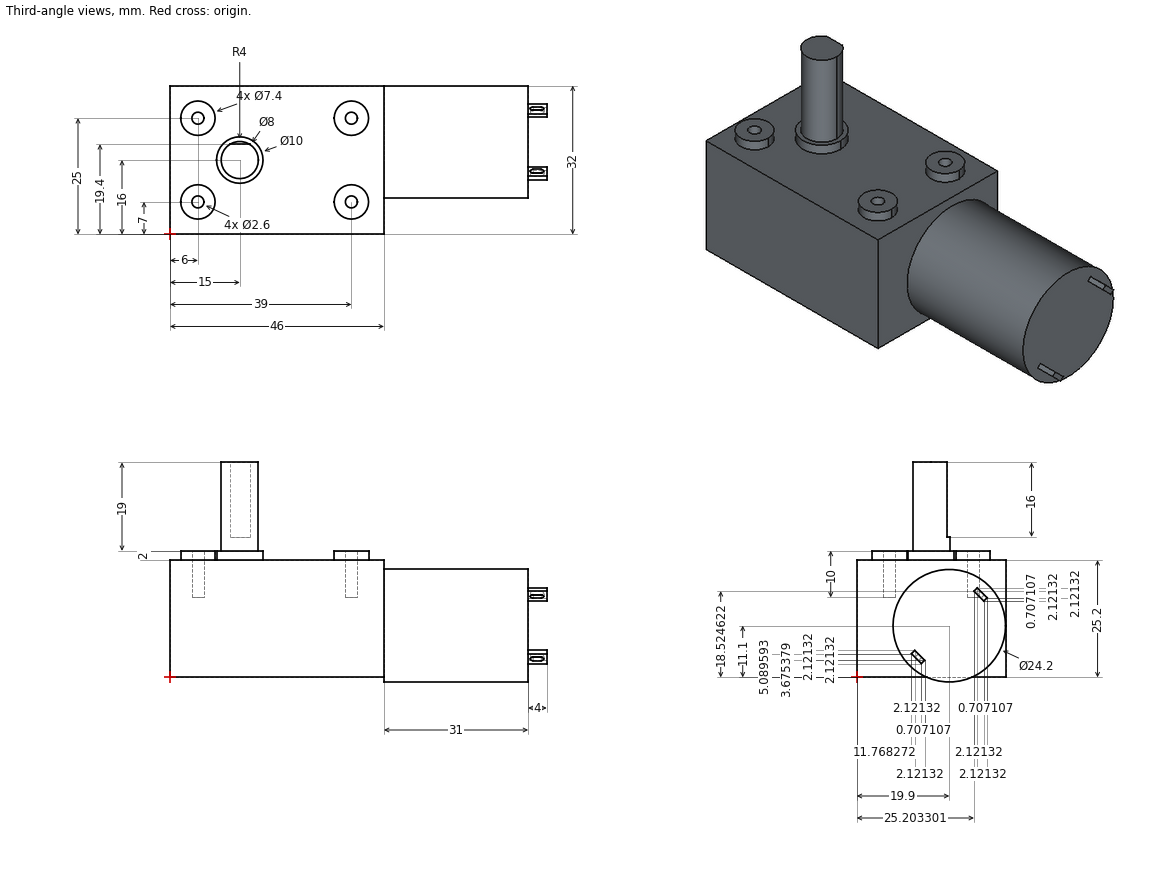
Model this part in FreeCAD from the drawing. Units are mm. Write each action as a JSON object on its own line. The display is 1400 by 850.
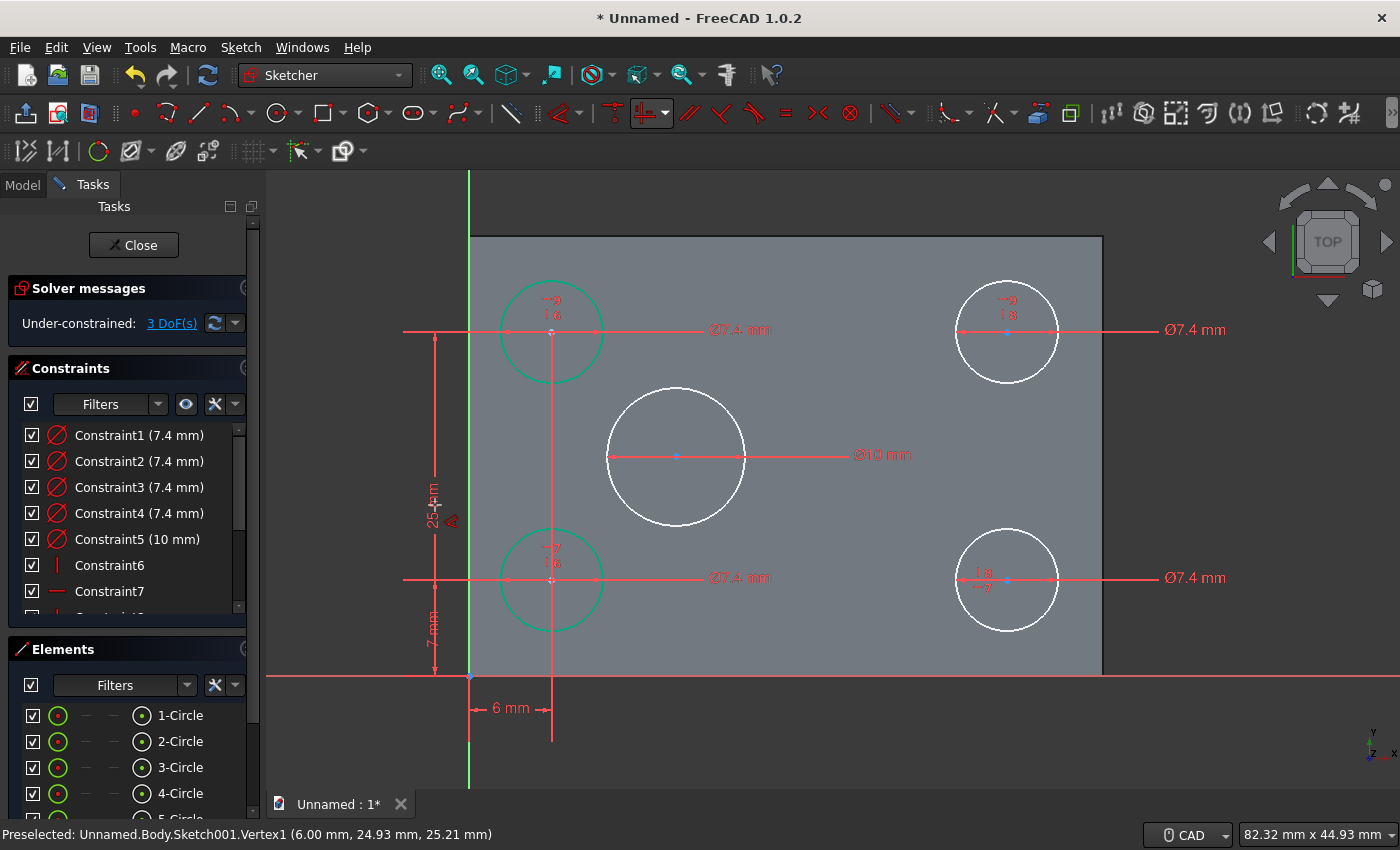
{"action": "left_click", "coordinate": [1007, 580]}
{"action": "left_click", "coordinate": [738, 710]}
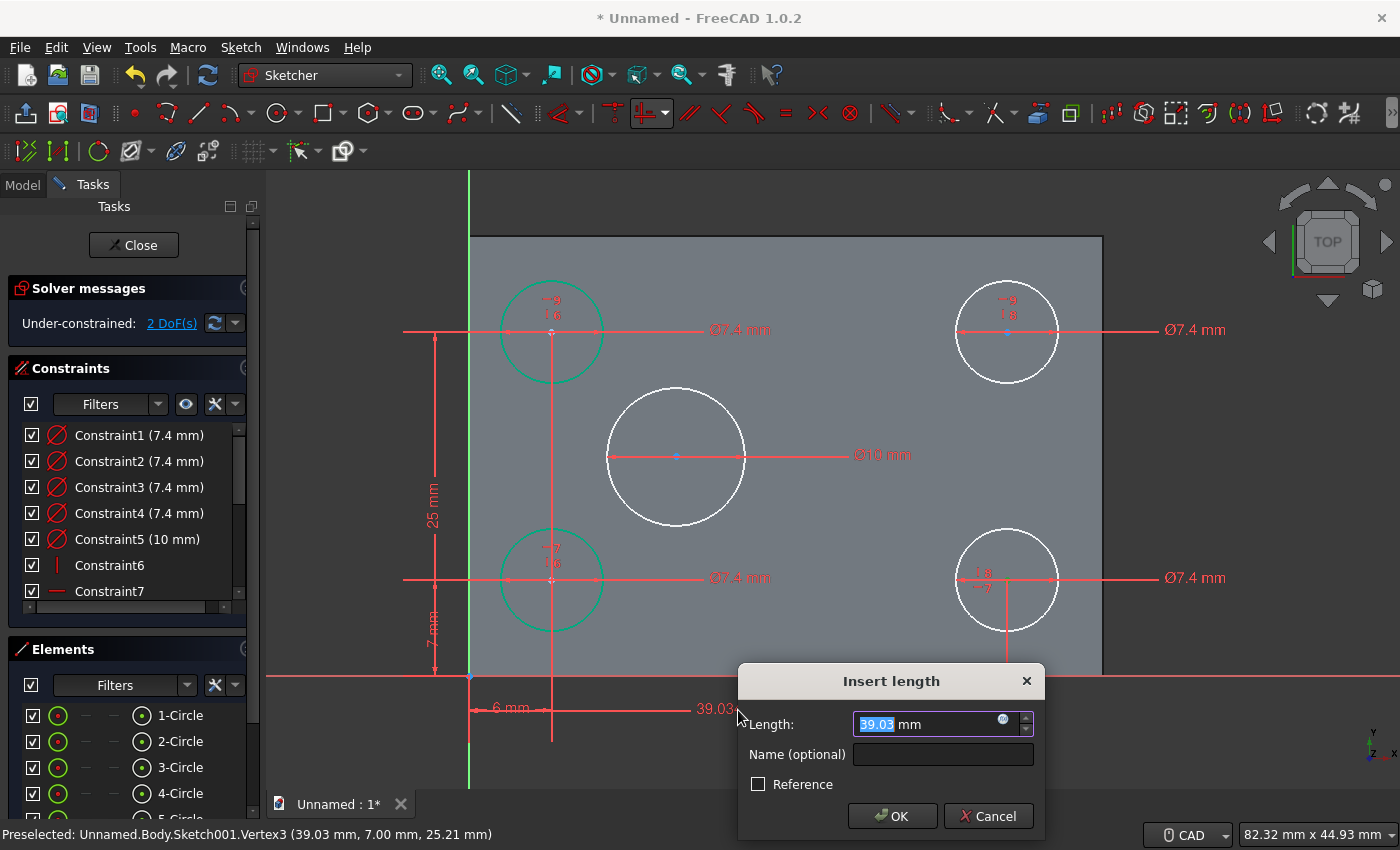
{"action": "type", "text": "39"}
{"action": "key", "text": "Return"}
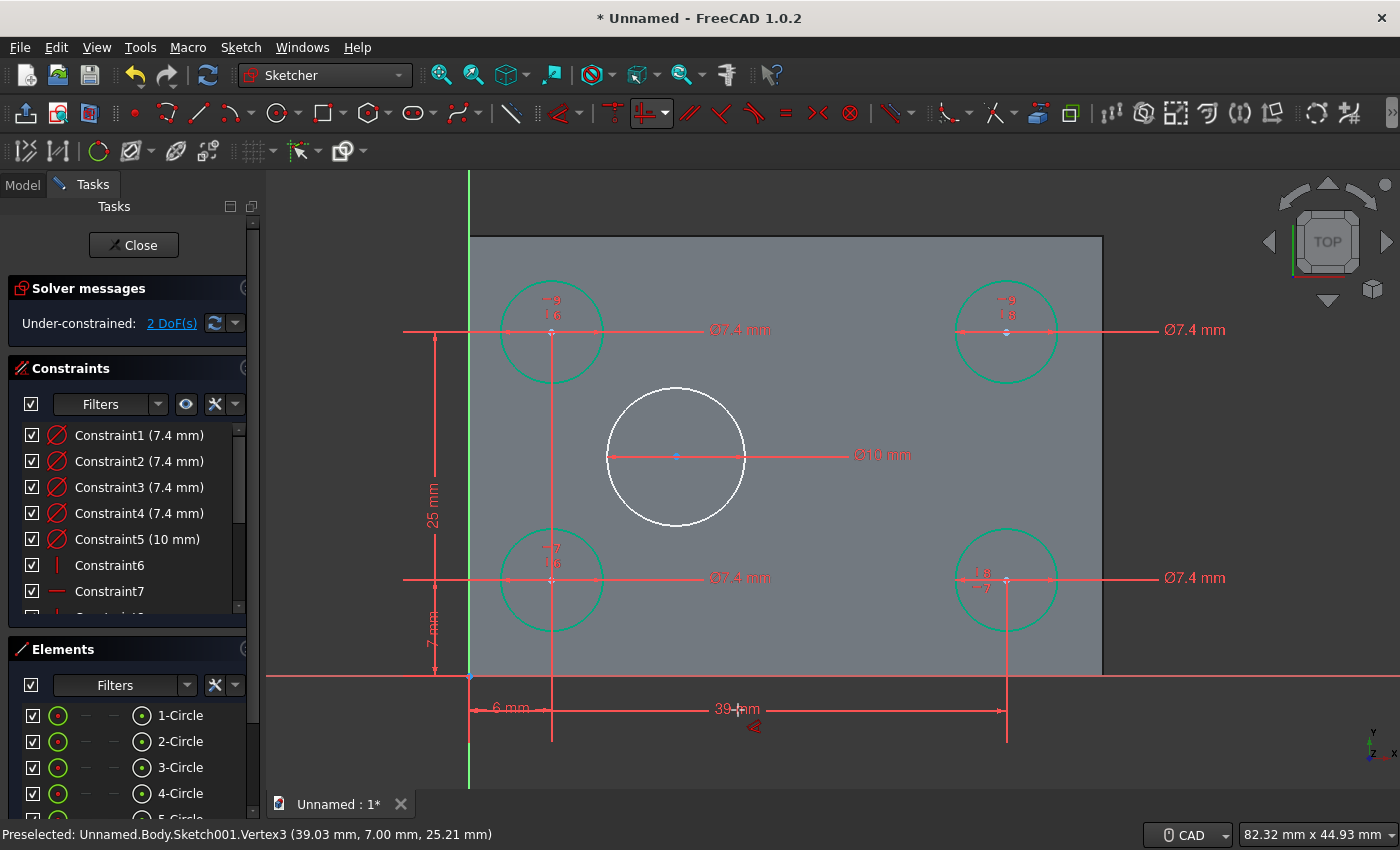
{"action": "left_click", "coordinate": [676, 457]}
{"action": "left_click", "coordinate": [620, 710]}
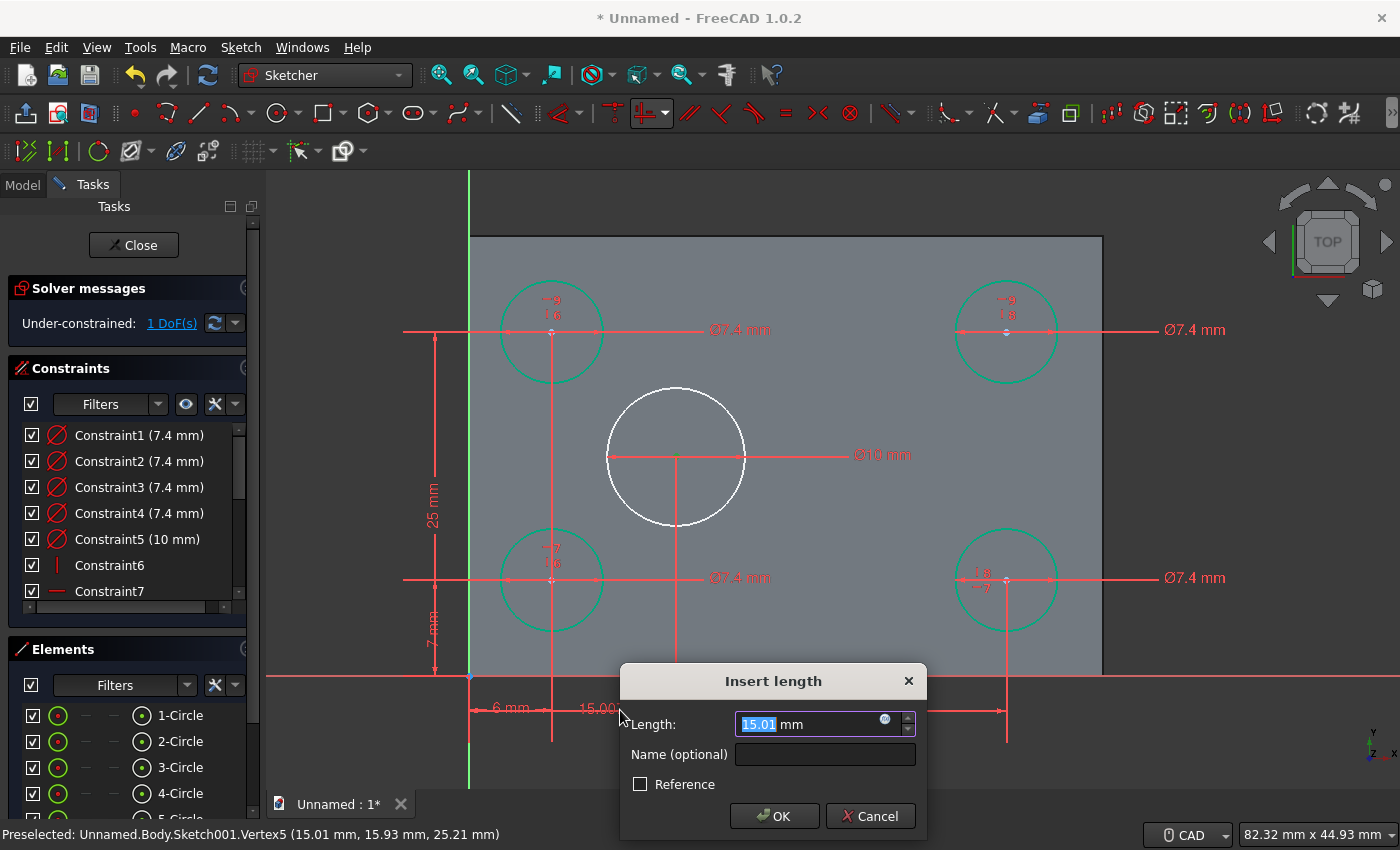
{"action": "type", "text": "15"}
{"action": "key", "text": "Return"}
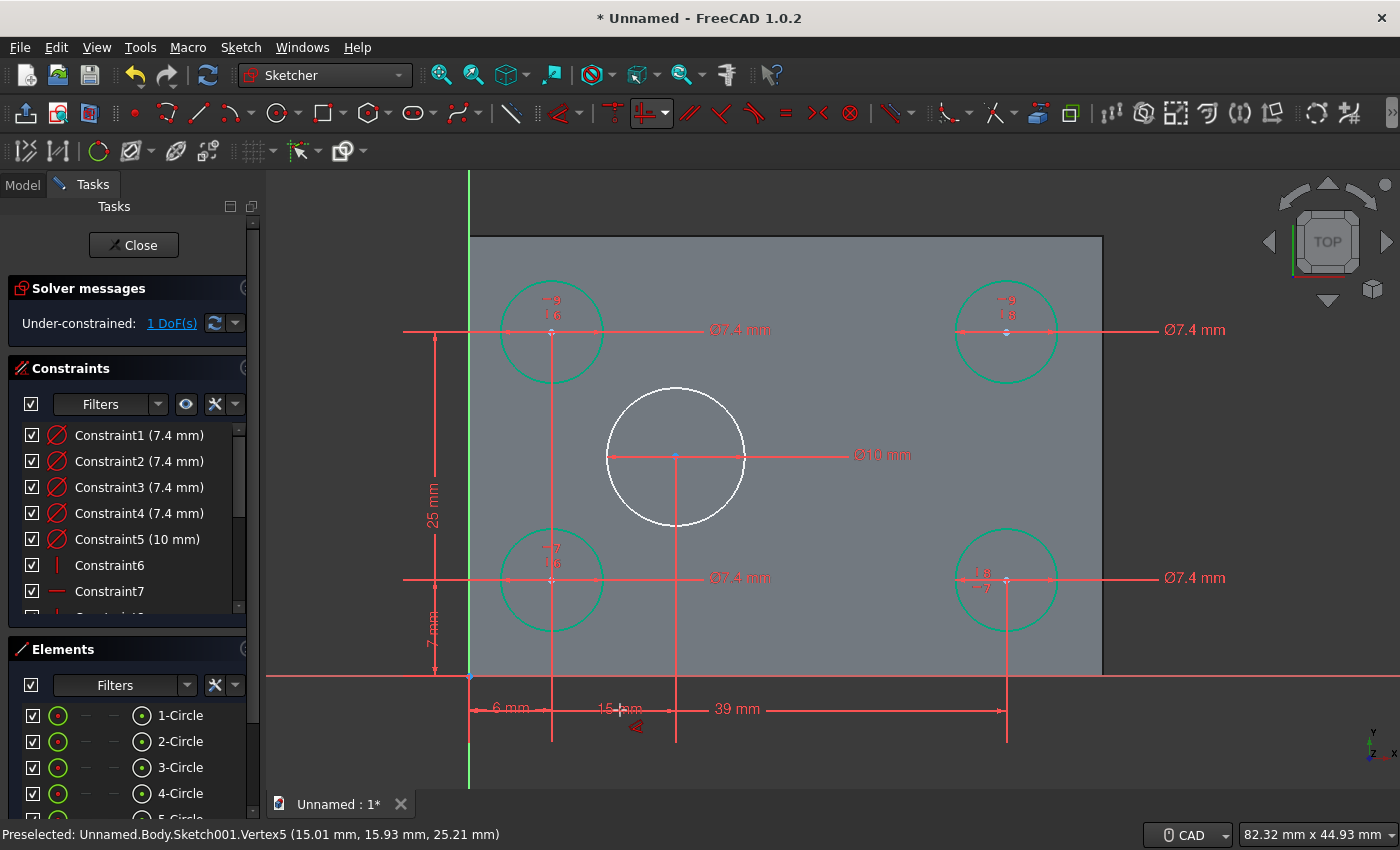
{"action": "left_click", "coordinate": [676, 457]}
{"action": "left_click", "coordinate": [435, 567]}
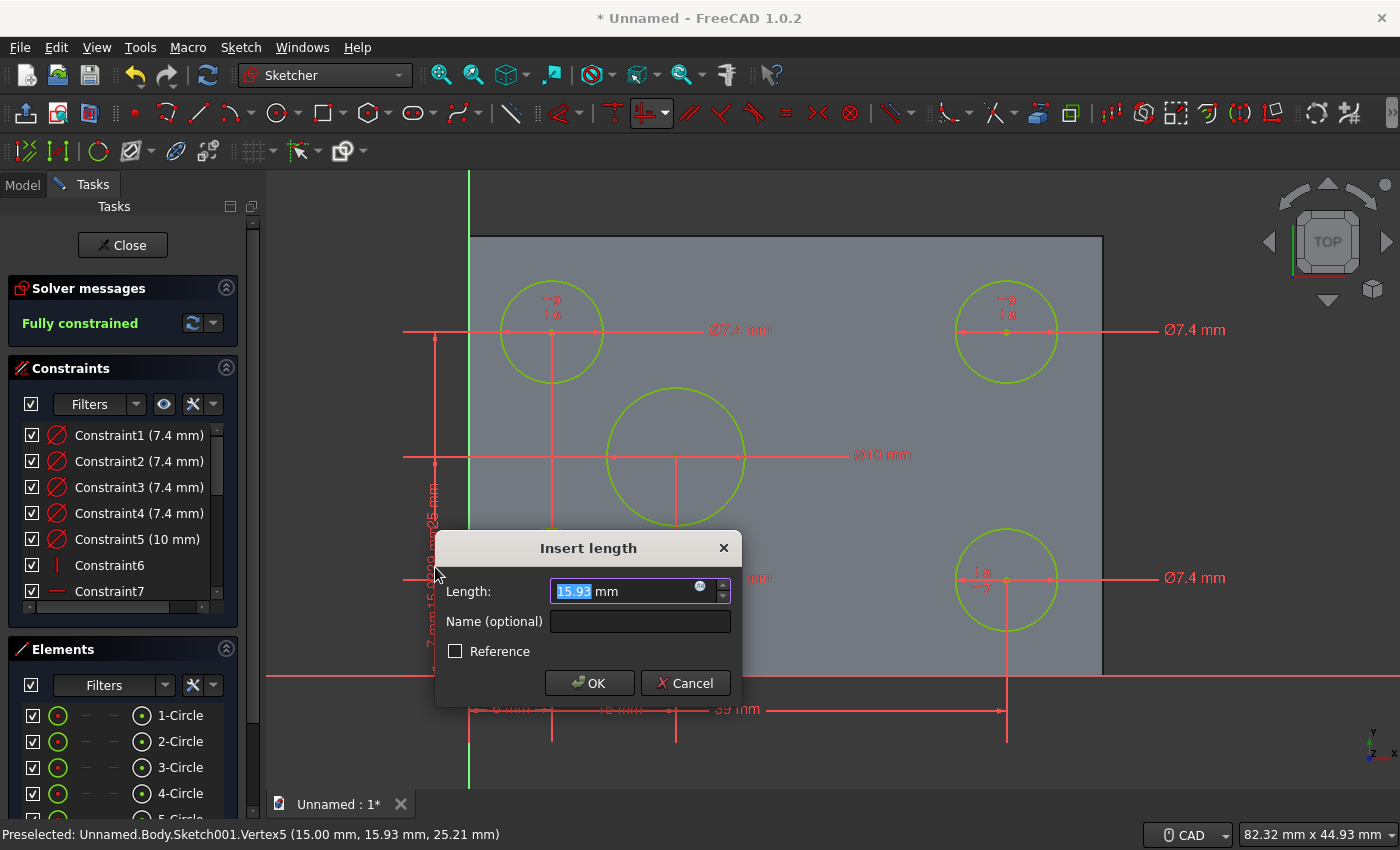
{"action": "type", "text": "16"}
{"action": "key", "text": "Return"}
{"action": "key", "text": "Escape"}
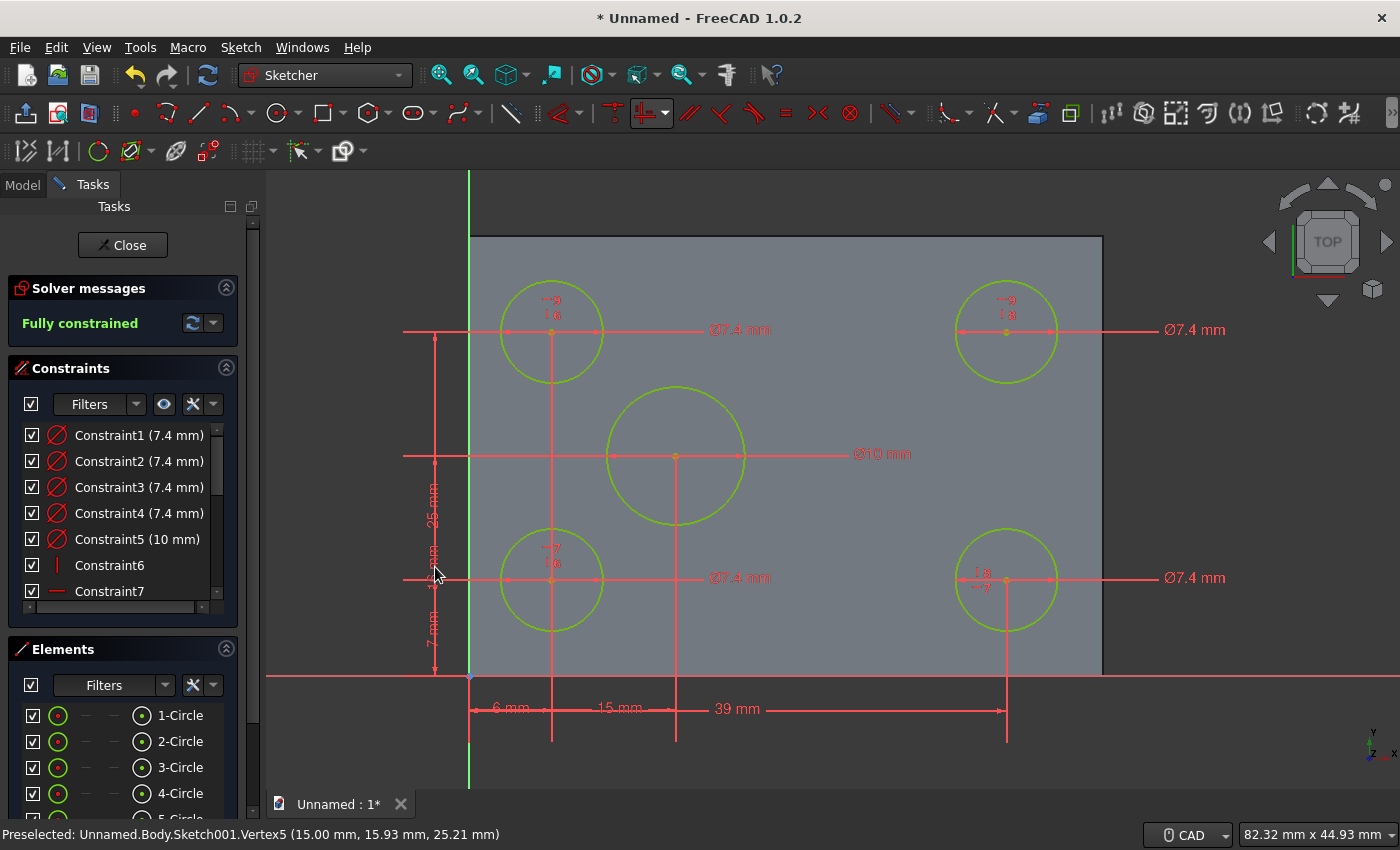
{"action": "left_click", "coordinate": [123, 245]}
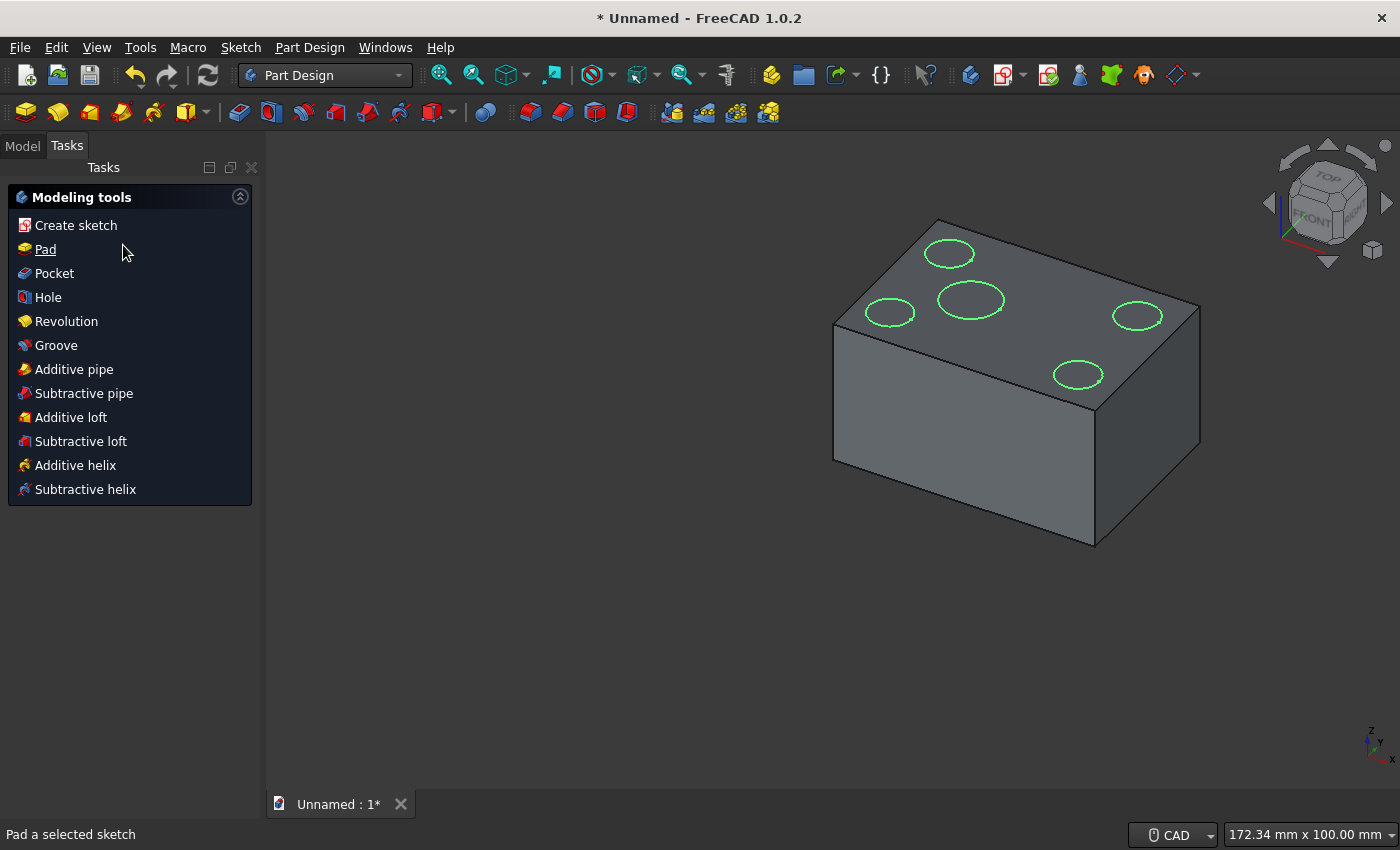
{"action": "left_click", "coordinate": [26, 112]}